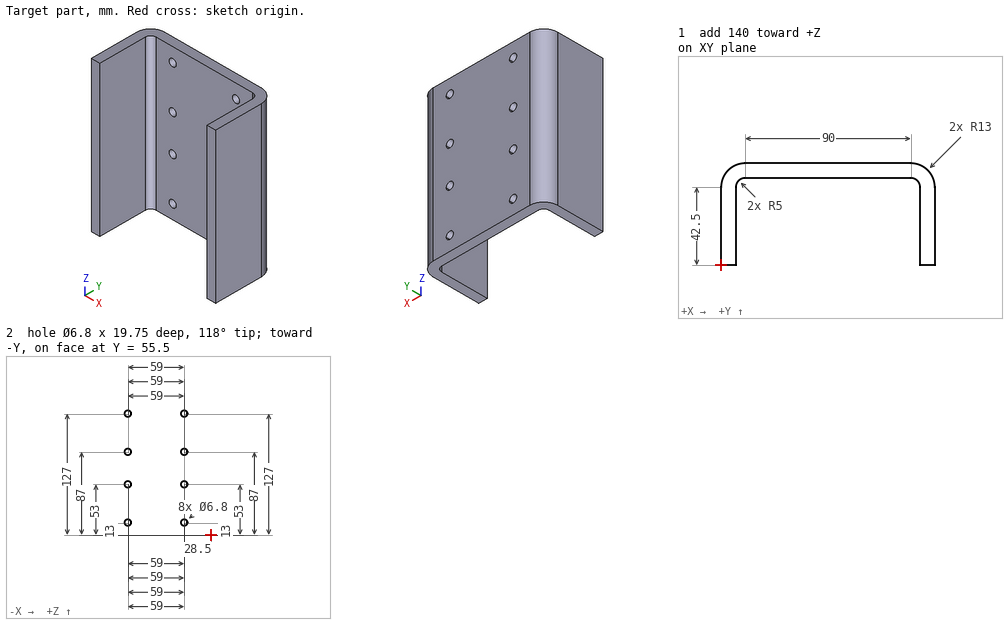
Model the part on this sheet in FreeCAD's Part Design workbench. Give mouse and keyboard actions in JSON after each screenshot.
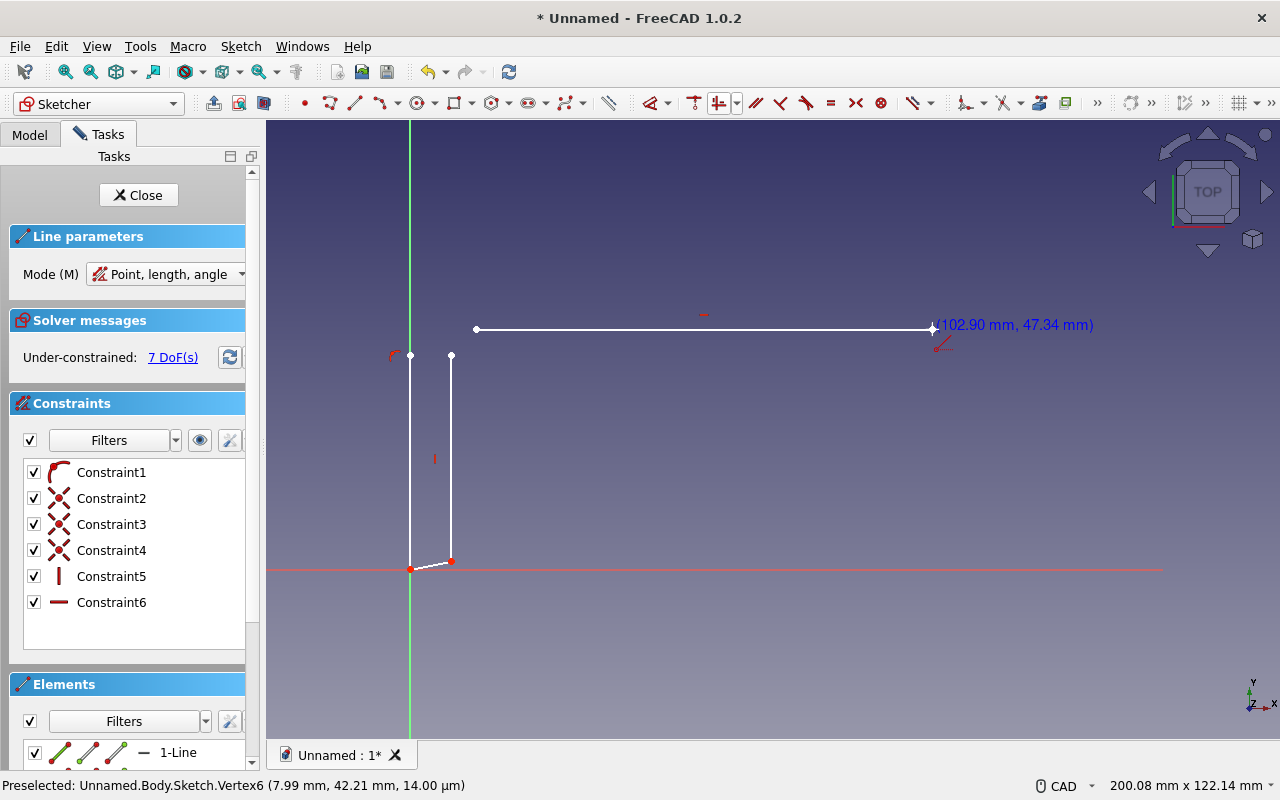
{"action": "key", "text": "g m"}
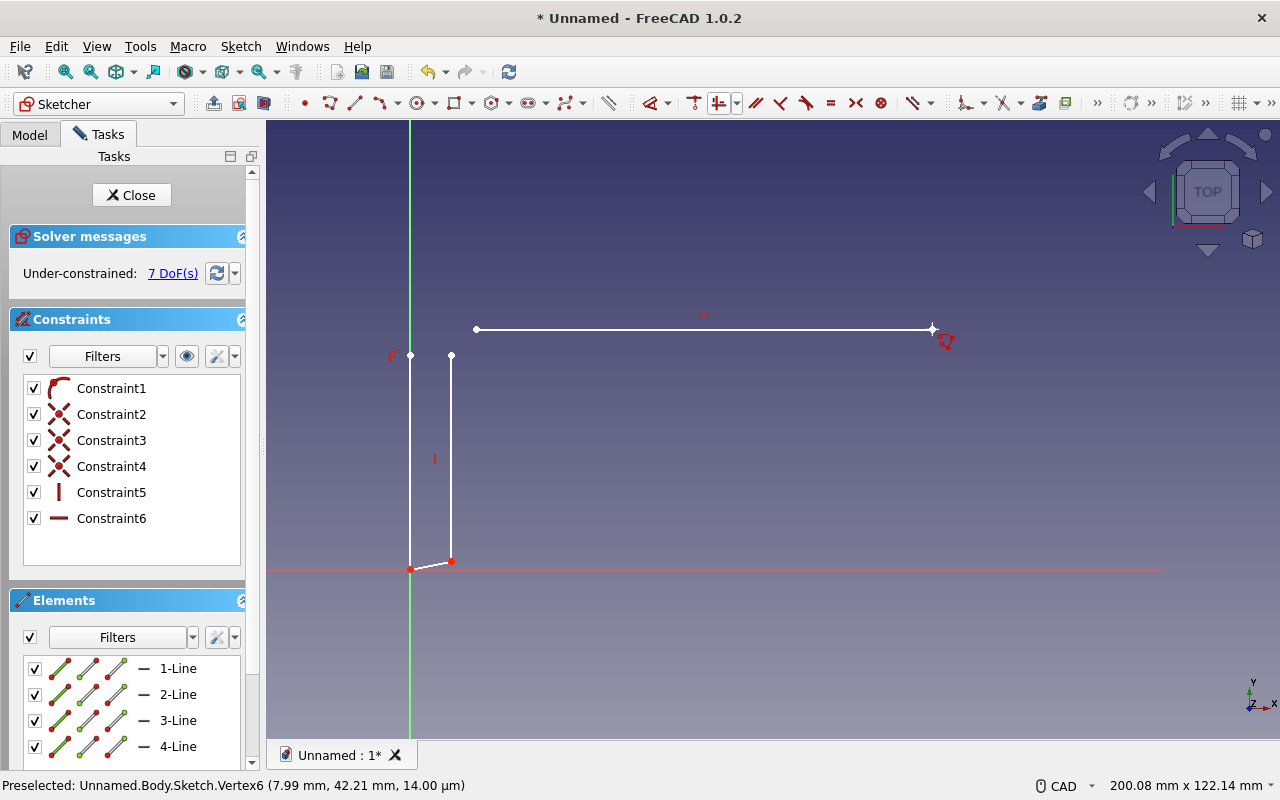
{"action": "left_click", "coordinate": [958, 355]}
{"action": "left_click", "coordinate": [958, 570]}
{"action": "left_click", "coordinate": [998, 561]}
{"action": "left_click", "coordinate": [998, 355]}
{"action": "right_click", "coordinate": [998, 355]}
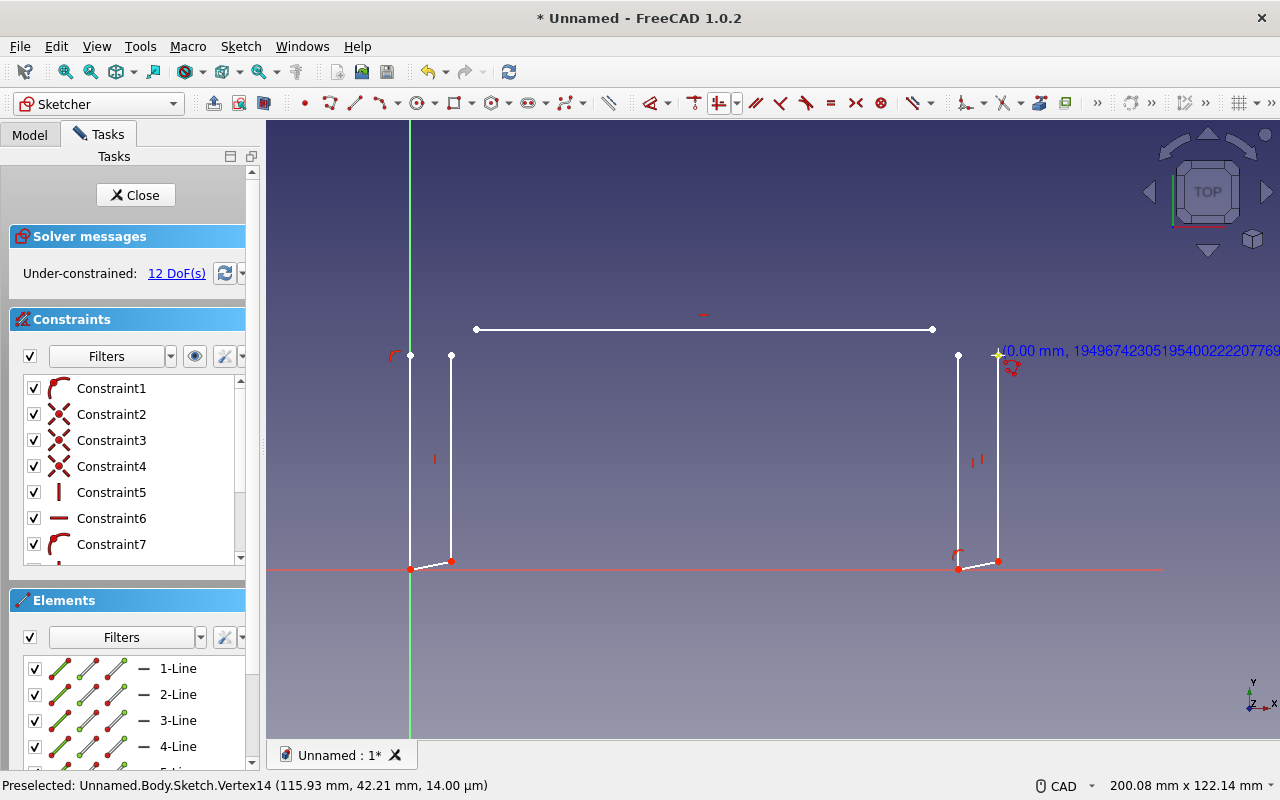
{"action": "left_click", "coordinate": [355, 104]}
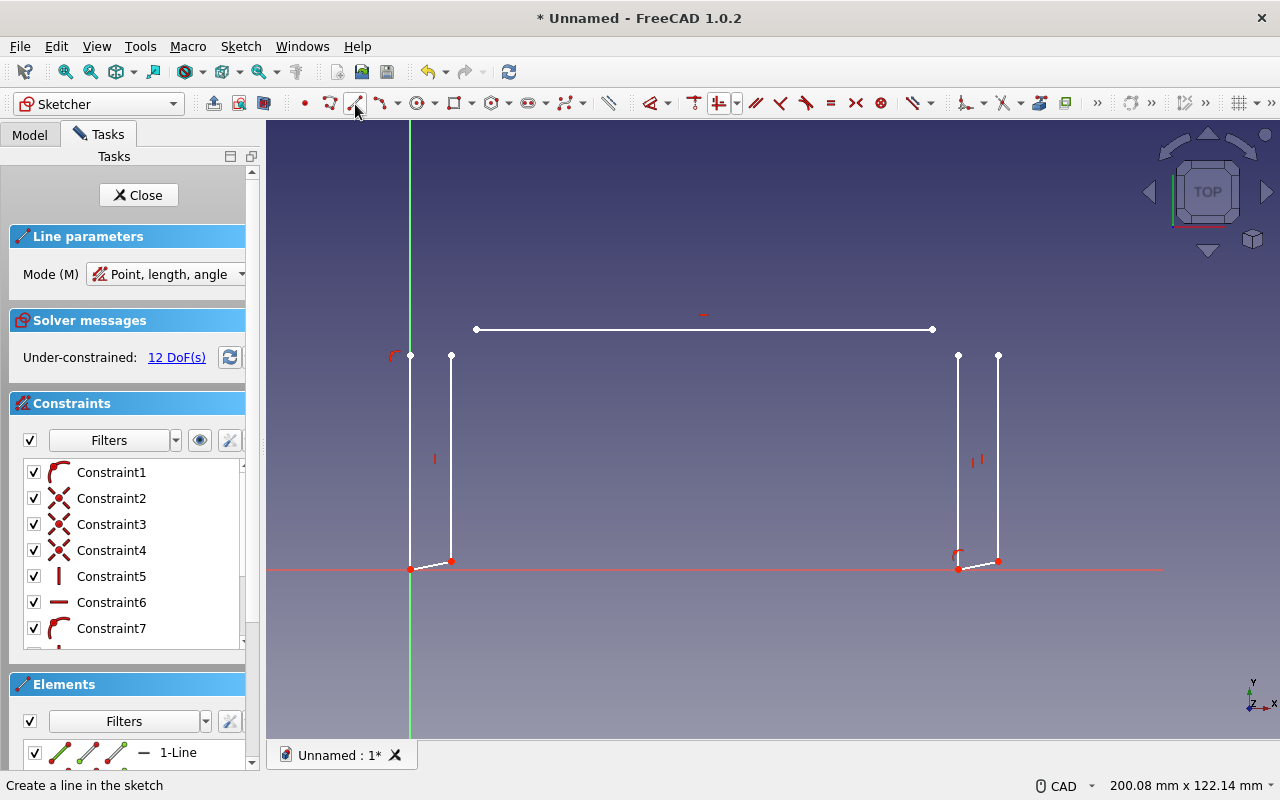
{"action": "left_click", "coordinate": [932, 289]}
{"action": "left_click", "coordinate": [476, 289]}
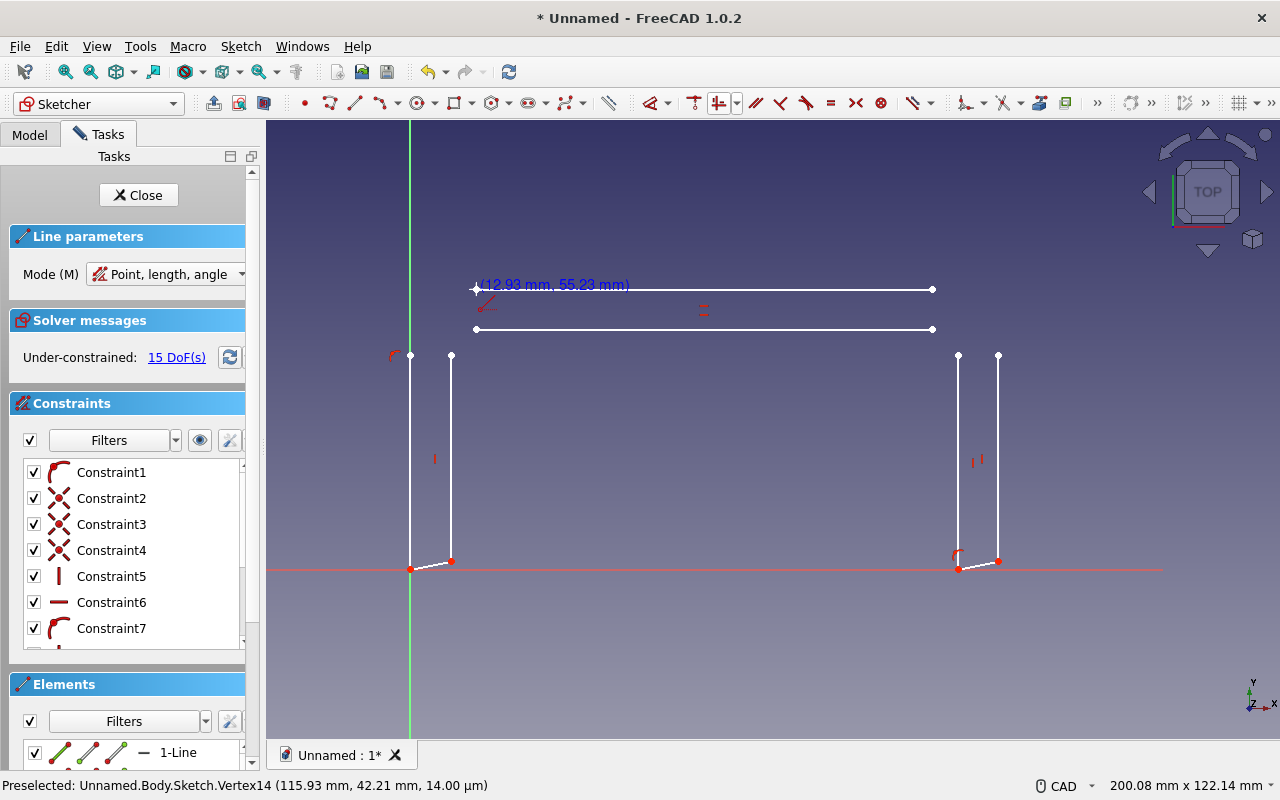
{"action": "key", "text": "g 3 a"}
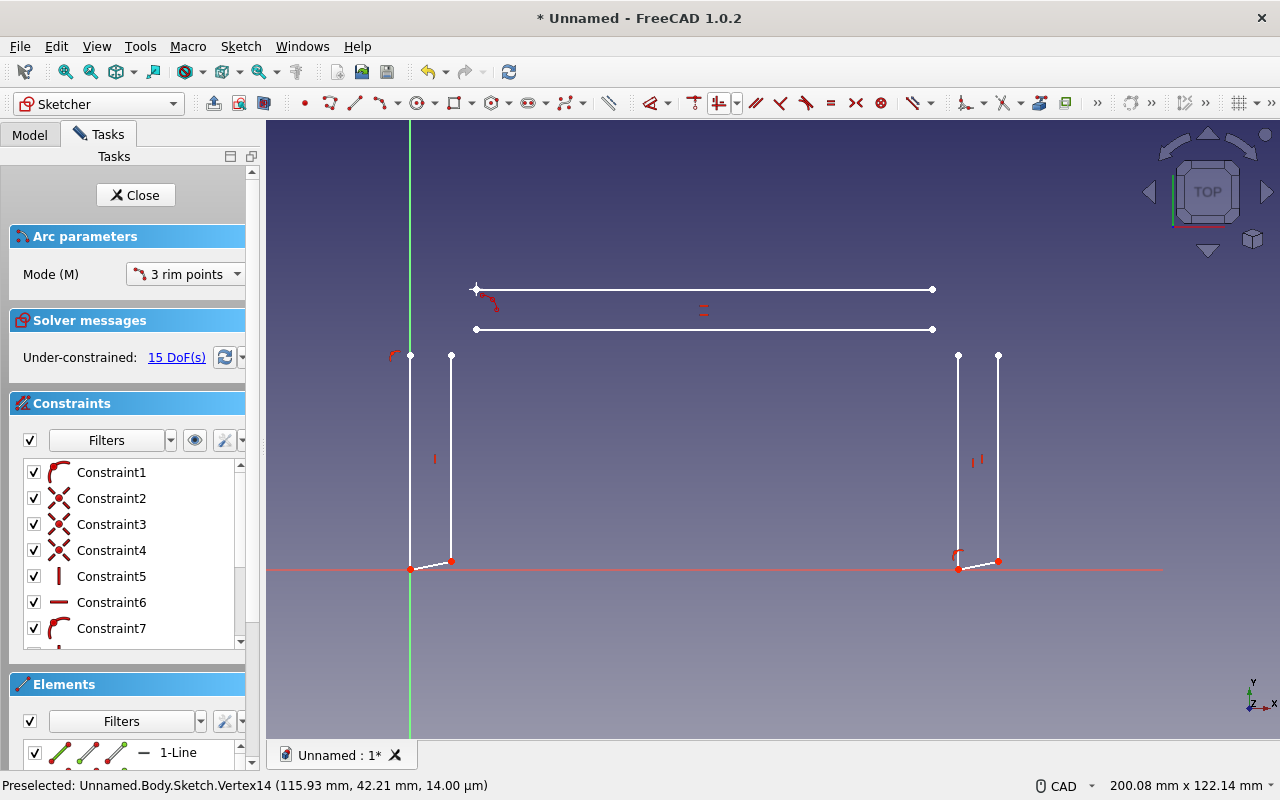
{"action": "left_click", "coordinate": [451, 356]}
{"action": "left_click", "coordinate": [476, 330]}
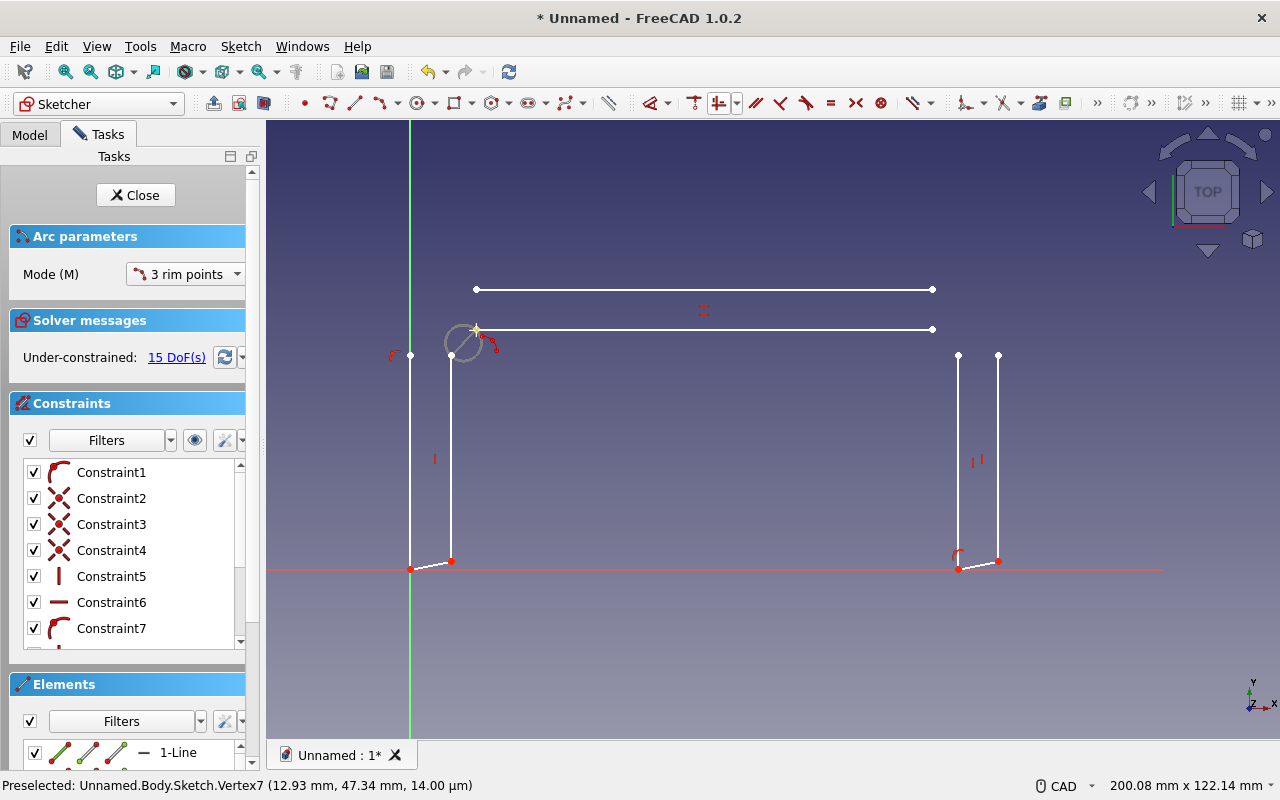
{"action": "scroll", "coordinate": [458, 337], "scroll_direction": "up", "scroll_amount": 4}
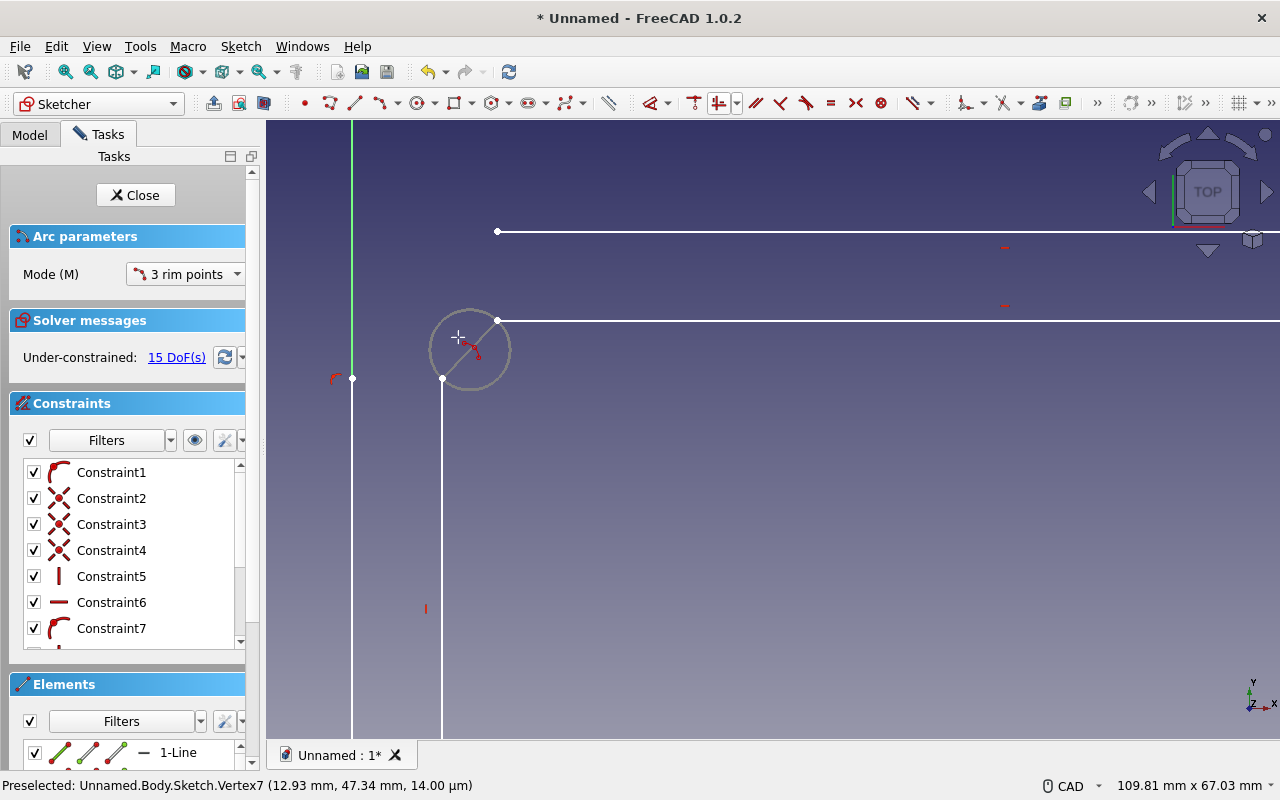
{"action": "left_click", "coordinate": [459, 336]}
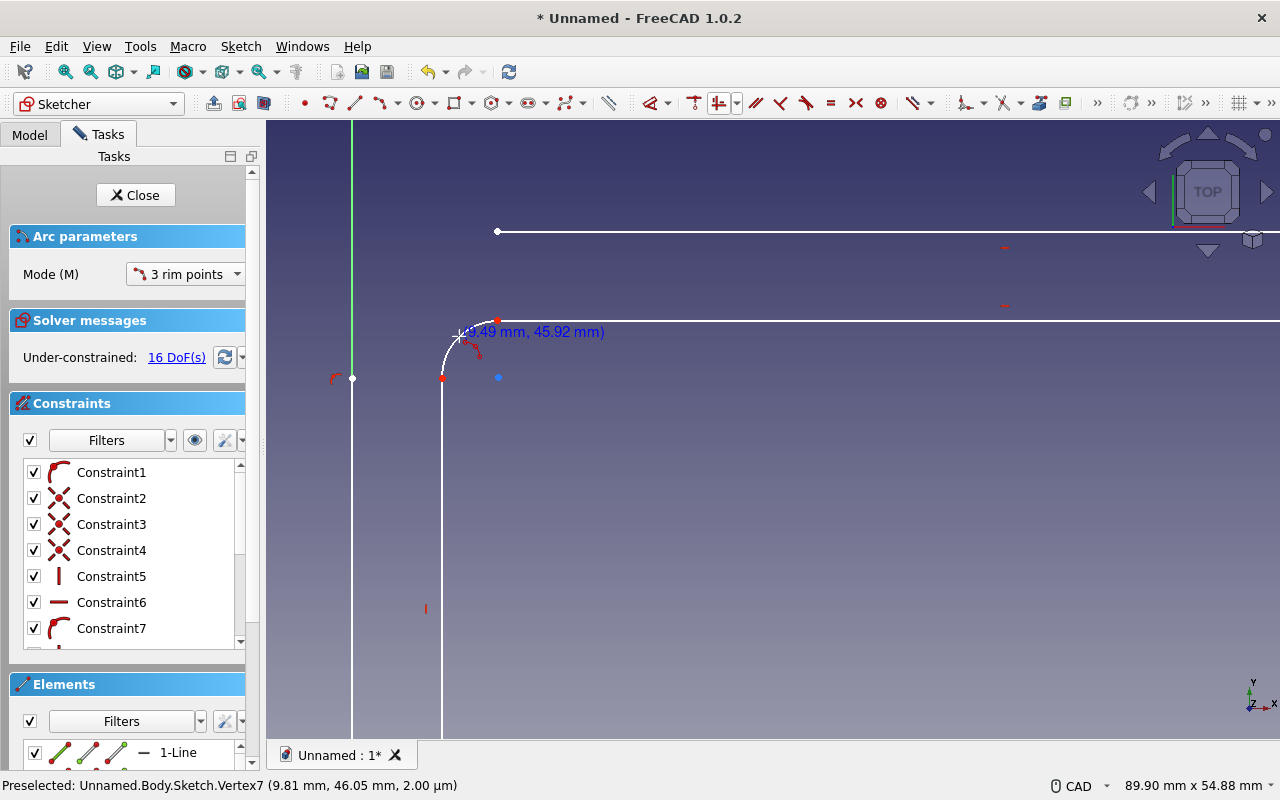
{"action": "scroll", "coordinate": [458, 338], "scroll_direction": "down", "scroll_amount": 4}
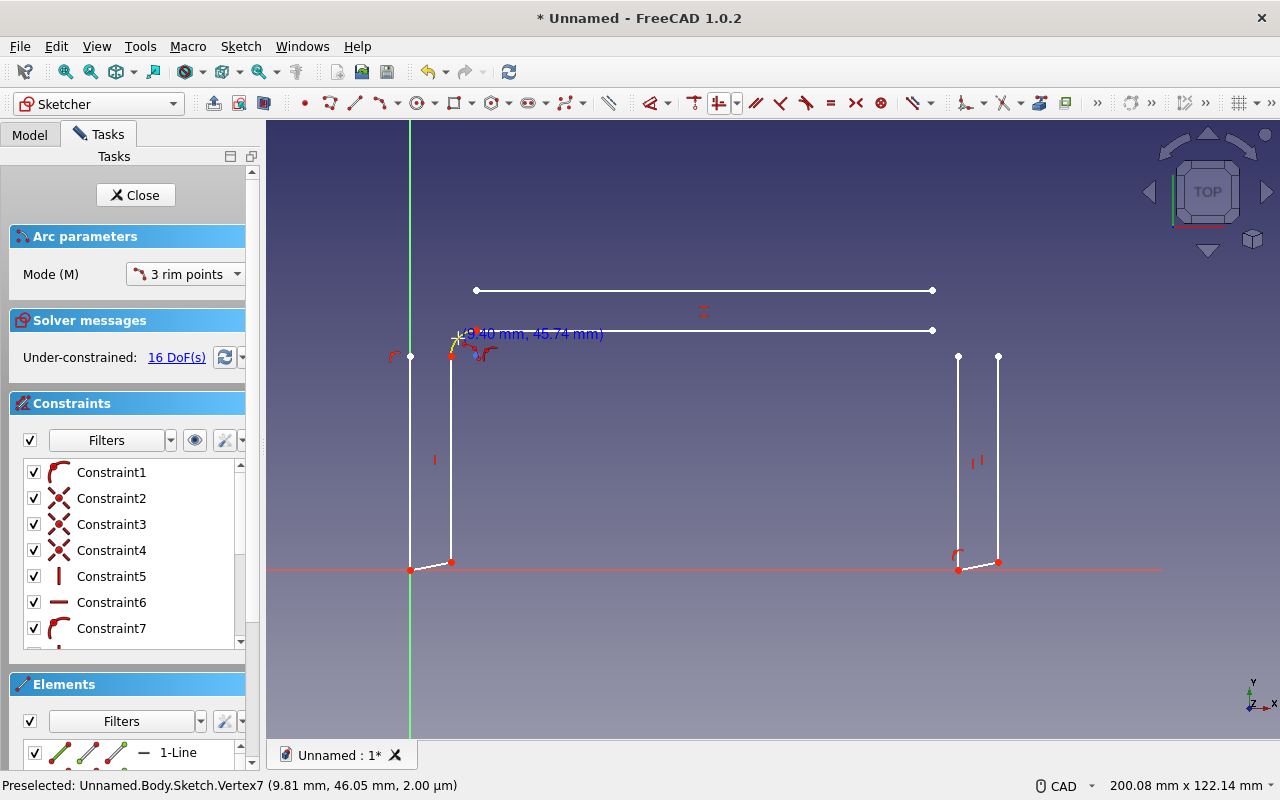
{"action": "left_click", "coordinate": [932, 331]}
{"action": "left_click", "coordinate": [958, 357]}